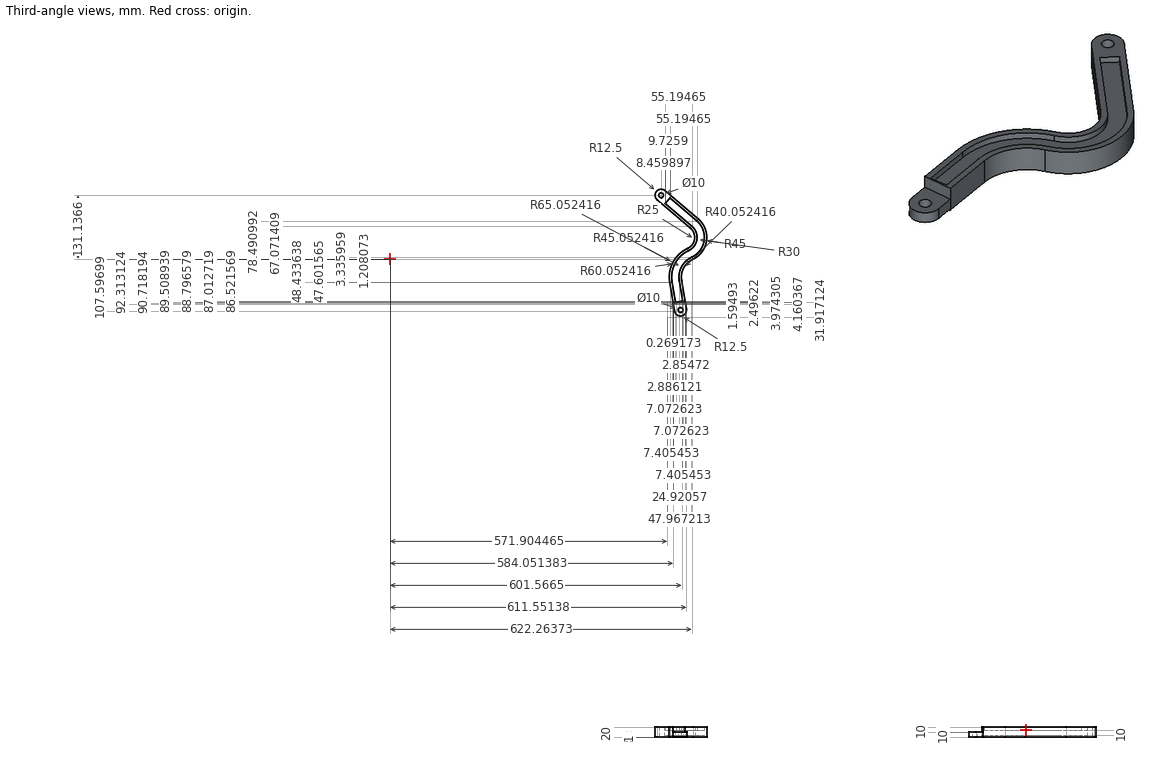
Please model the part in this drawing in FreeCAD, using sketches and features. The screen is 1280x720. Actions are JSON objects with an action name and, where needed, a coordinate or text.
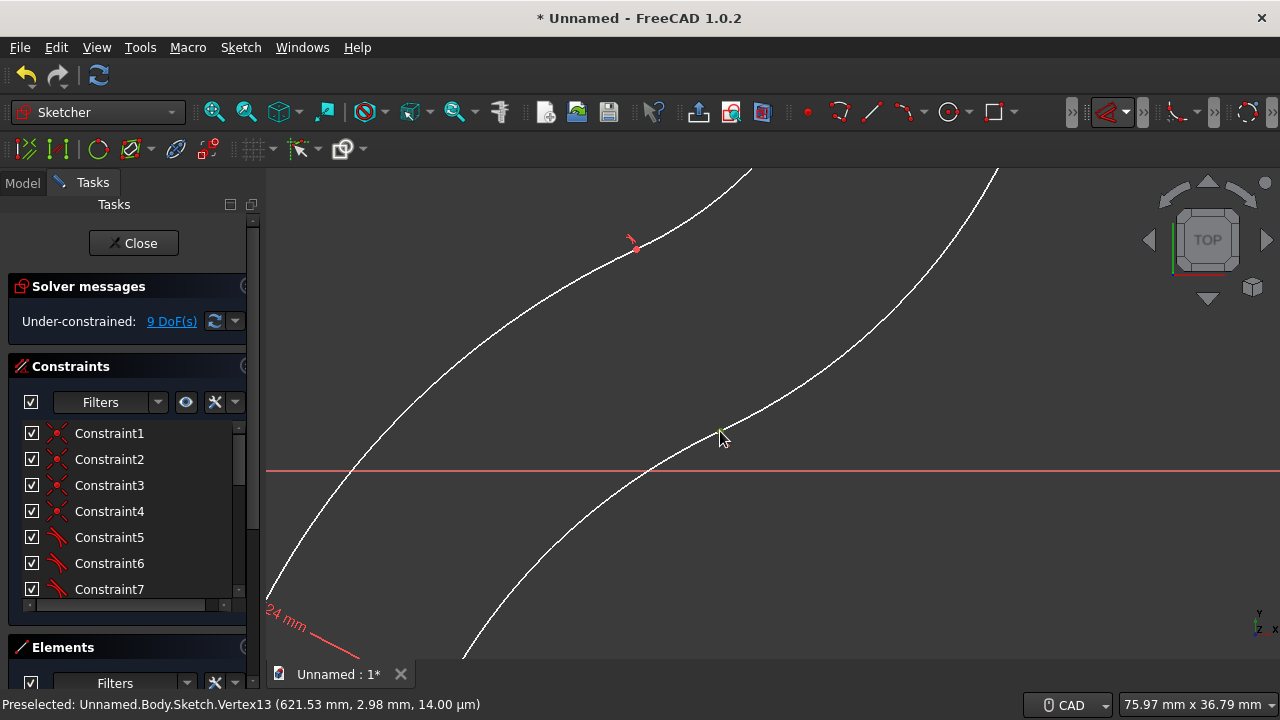
{"action": "key", "text": "i"}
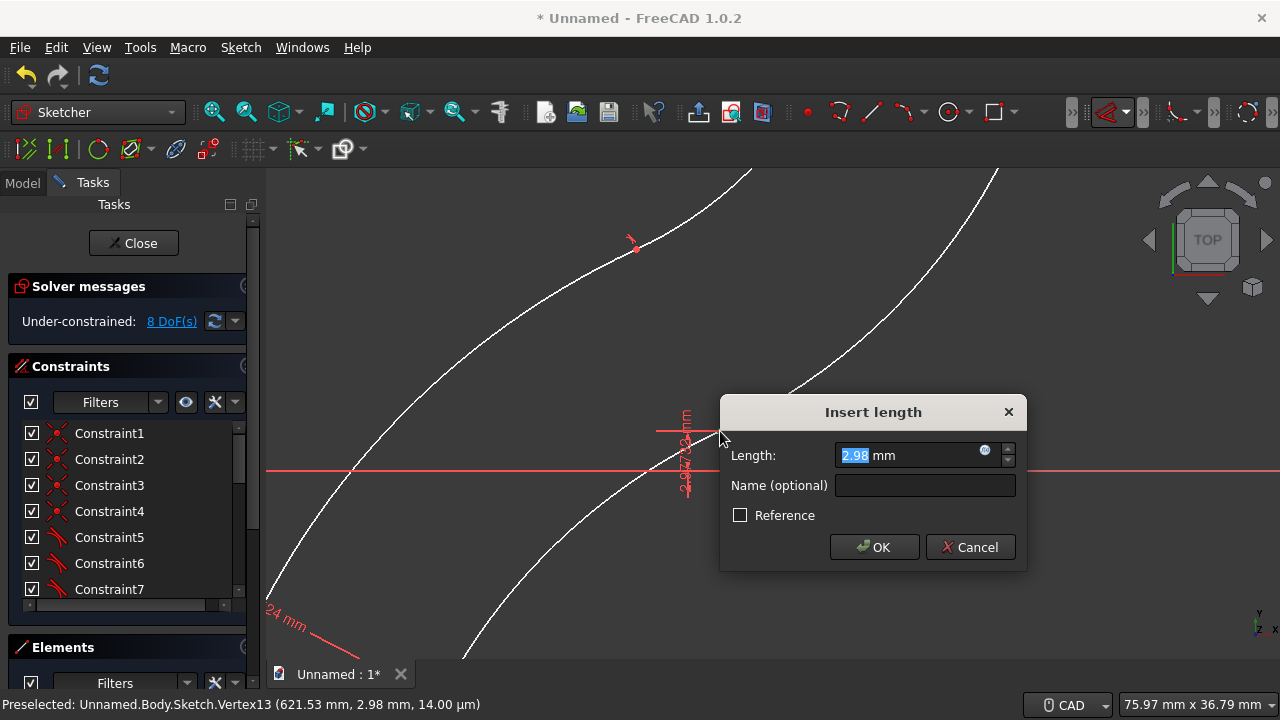
{"action": "type", "text": "3.335959"}
{"action": "key", "text": "Return"}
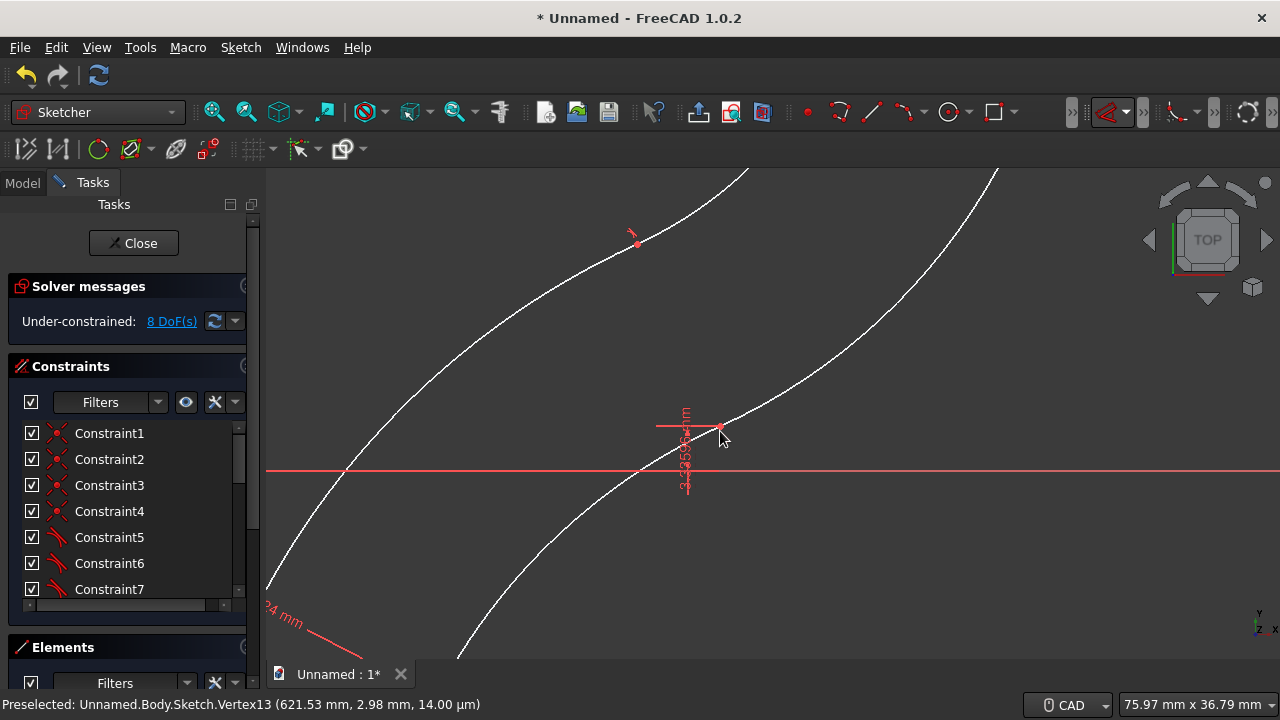
{"action": "scroll", "coordinate": [725, 436], "scroll_direction": "down", "scroll_amount": 11}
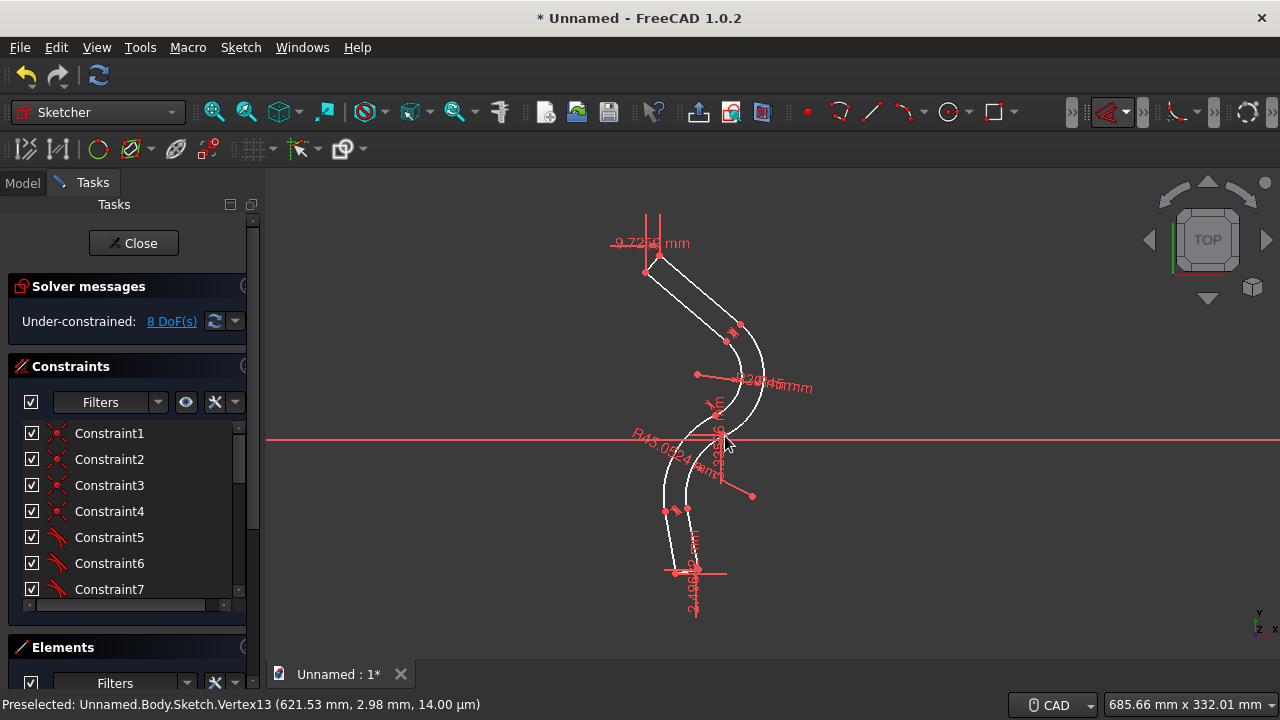
{"action": "scroll", "coordinate": [668, 530], "scroll_direction": "up", "scroll_amount": 7}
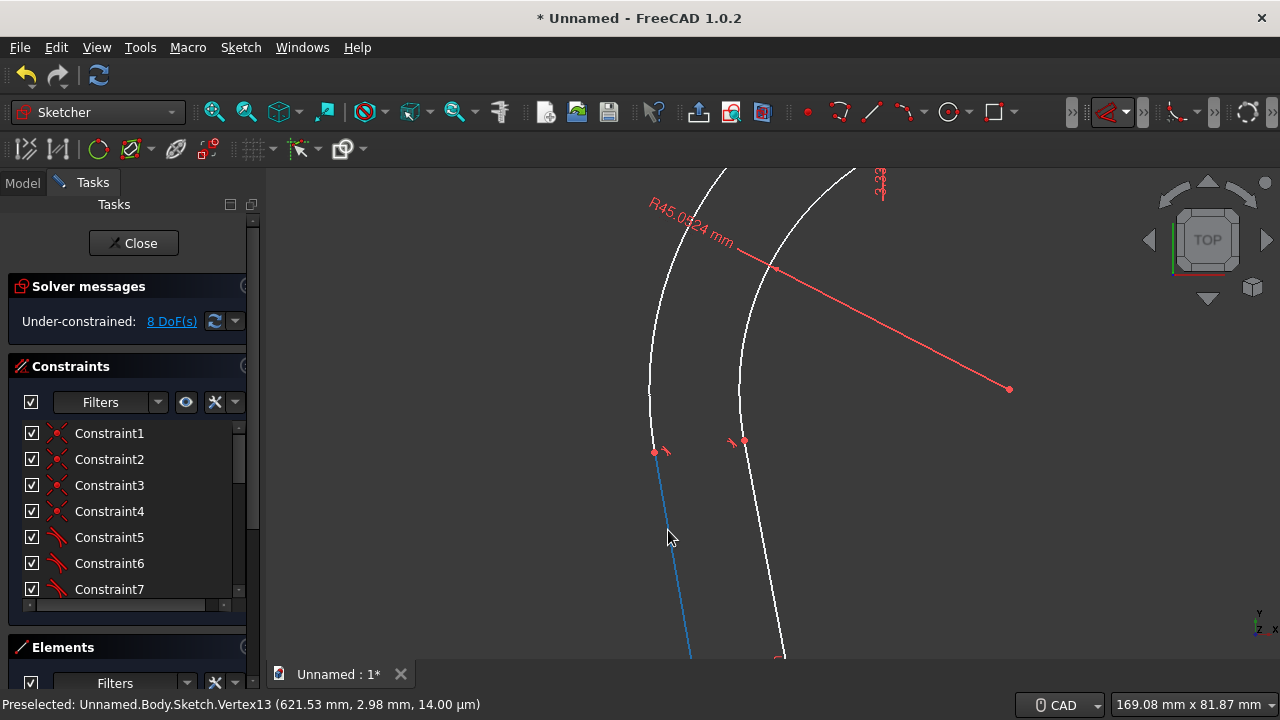
{"action": "left_click", "coordinate": [668, 528]}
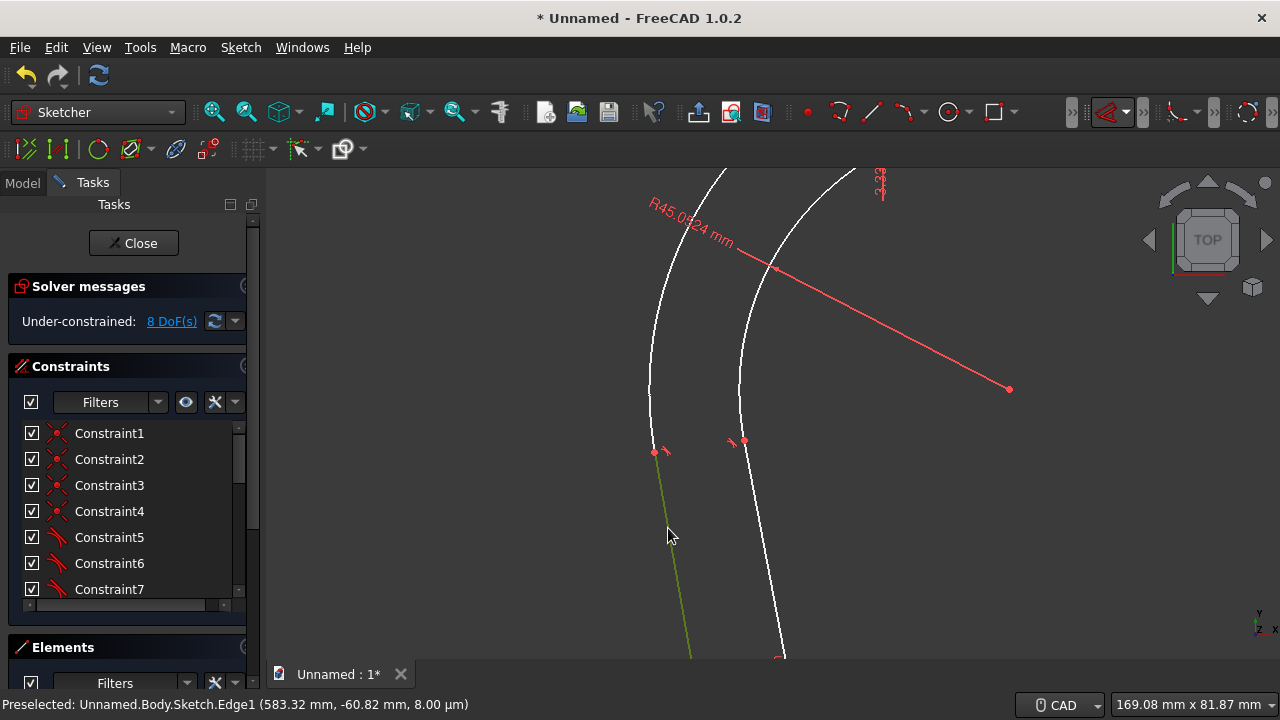
{"action": "key", "text": "l"}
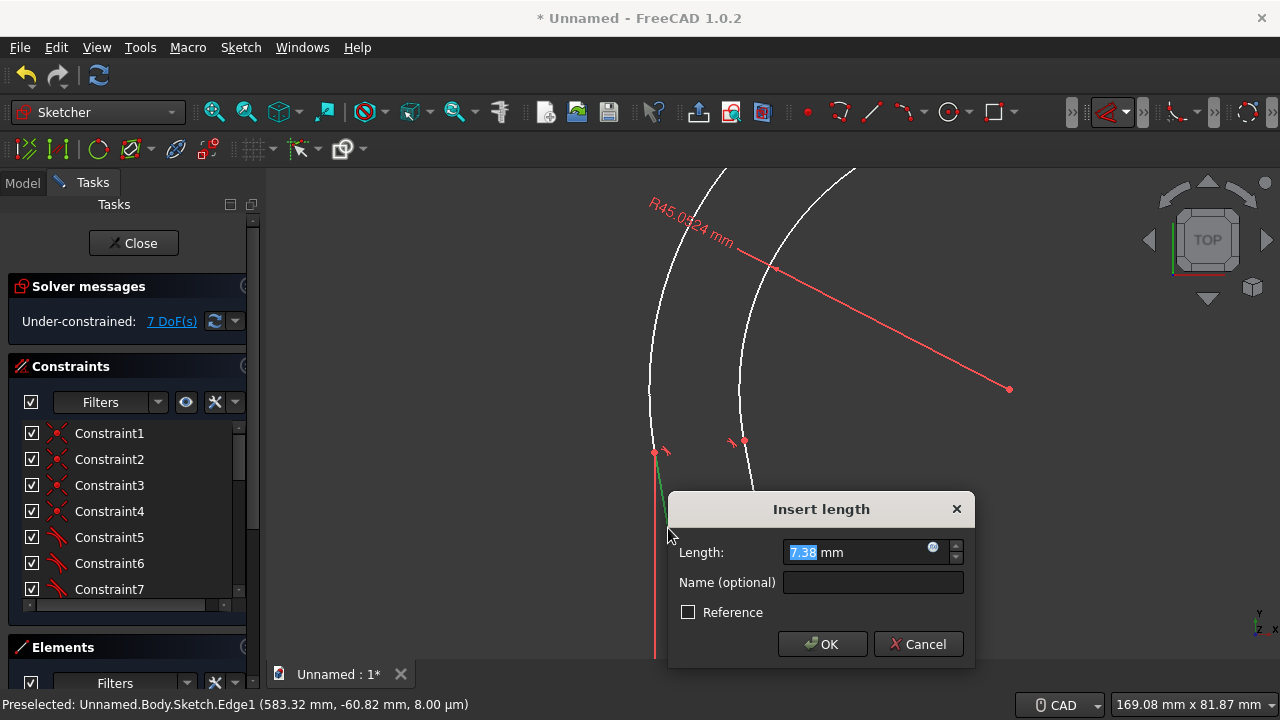
{"action": "type", "text": "7.072623"}
{"action": "key", "text": "Return"}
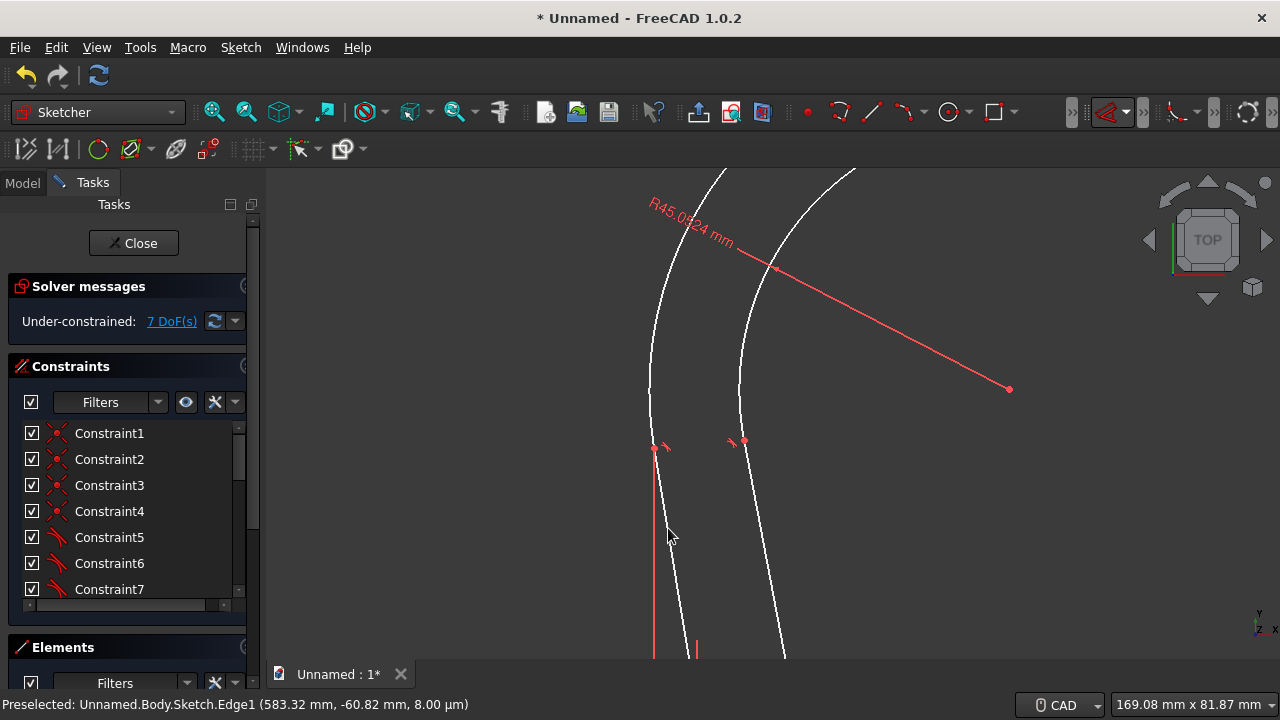
{"action": "left_click", "coordinate": [777, 615]}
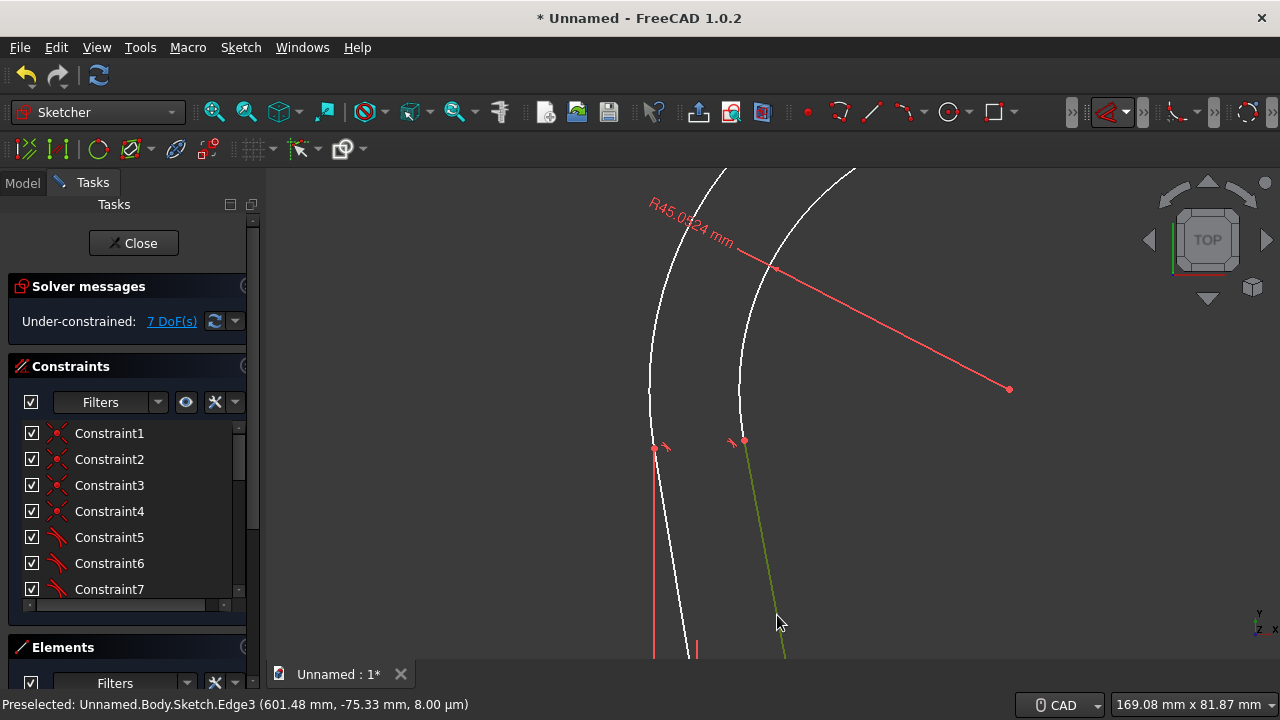
{"action": "left_click", "coordinate": [1128, 112]}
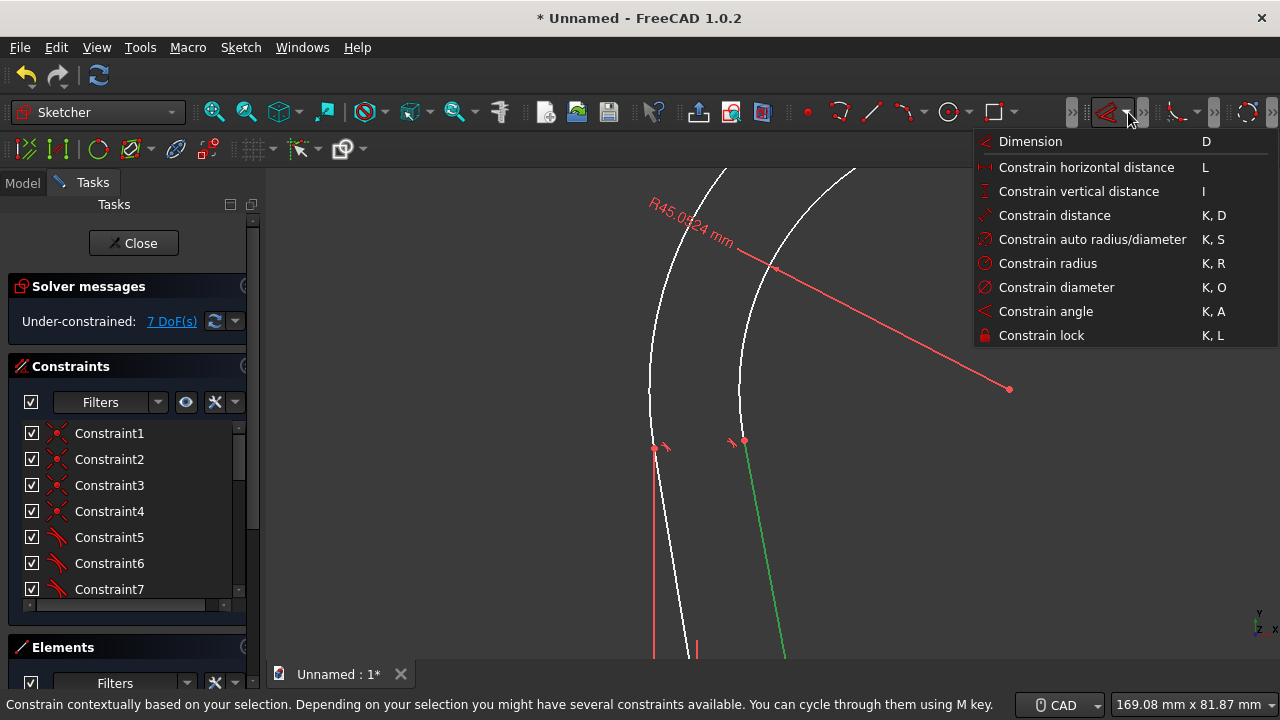
{"action": "left_click", "coordinate": [1126, 167]}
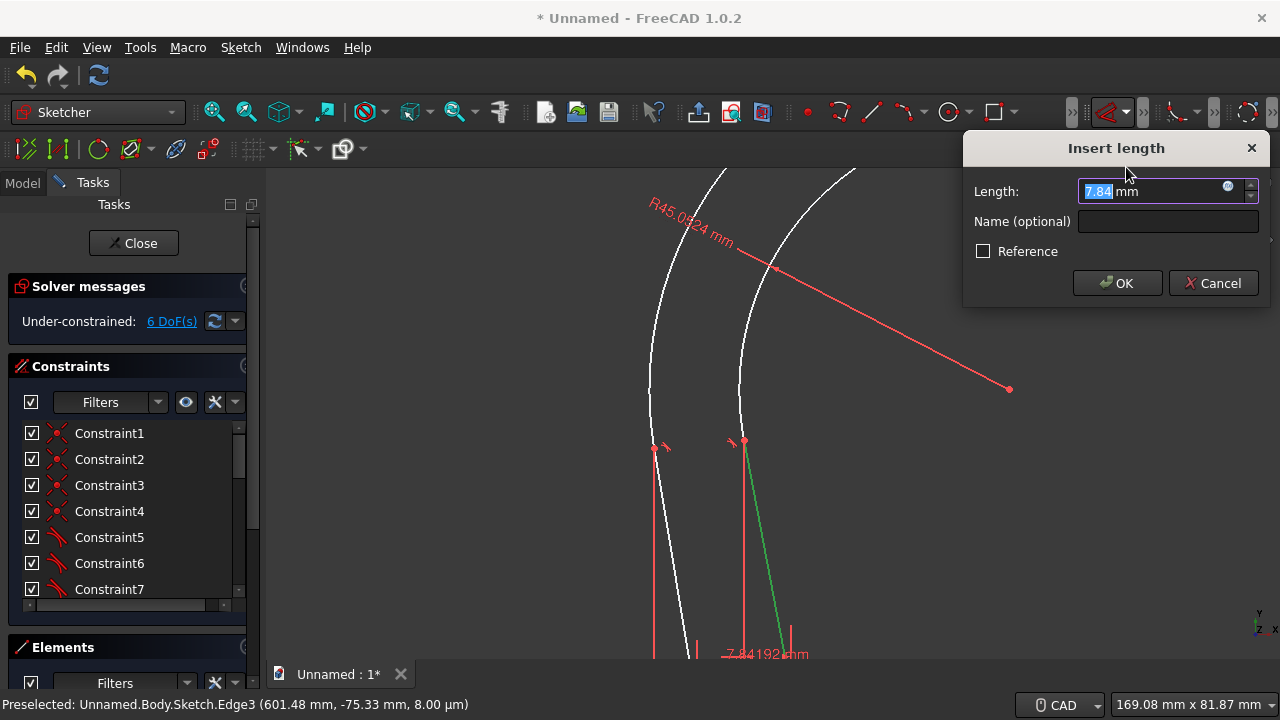
{"action": "type", "text": "7.072623"}
{"action": "key", "text": "Return"}